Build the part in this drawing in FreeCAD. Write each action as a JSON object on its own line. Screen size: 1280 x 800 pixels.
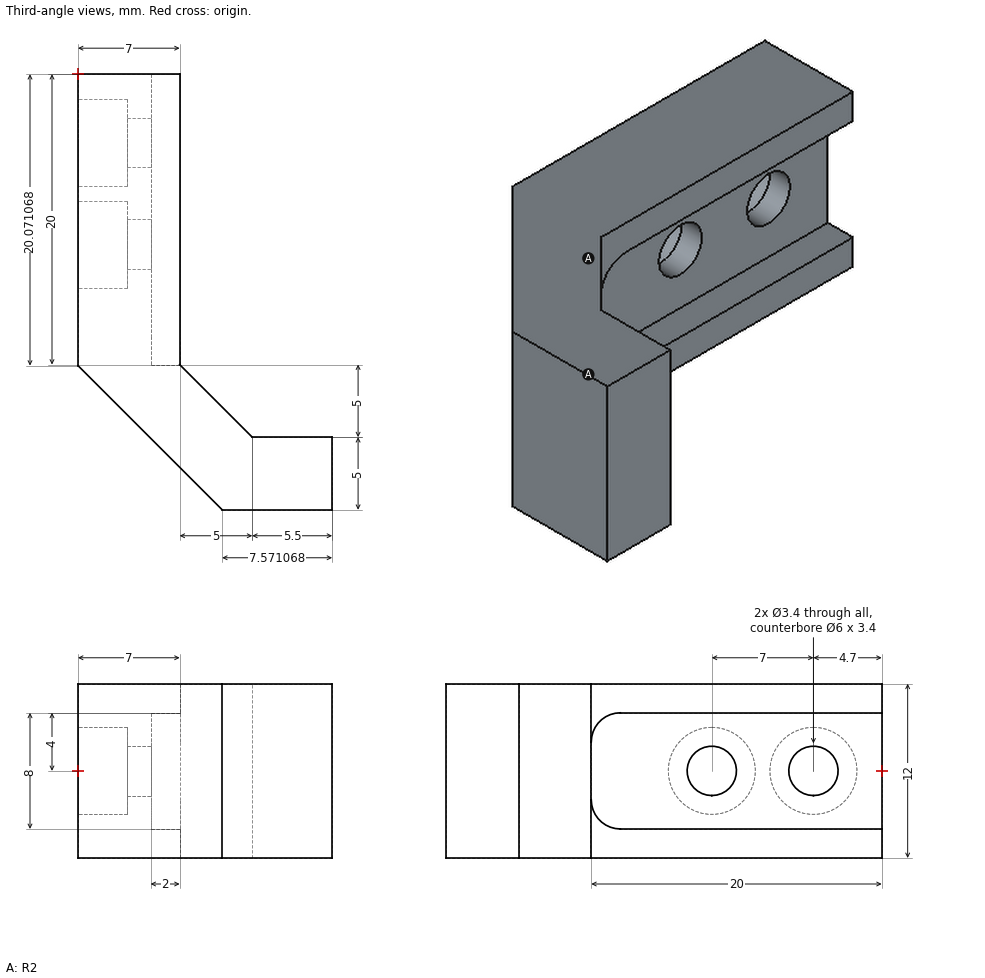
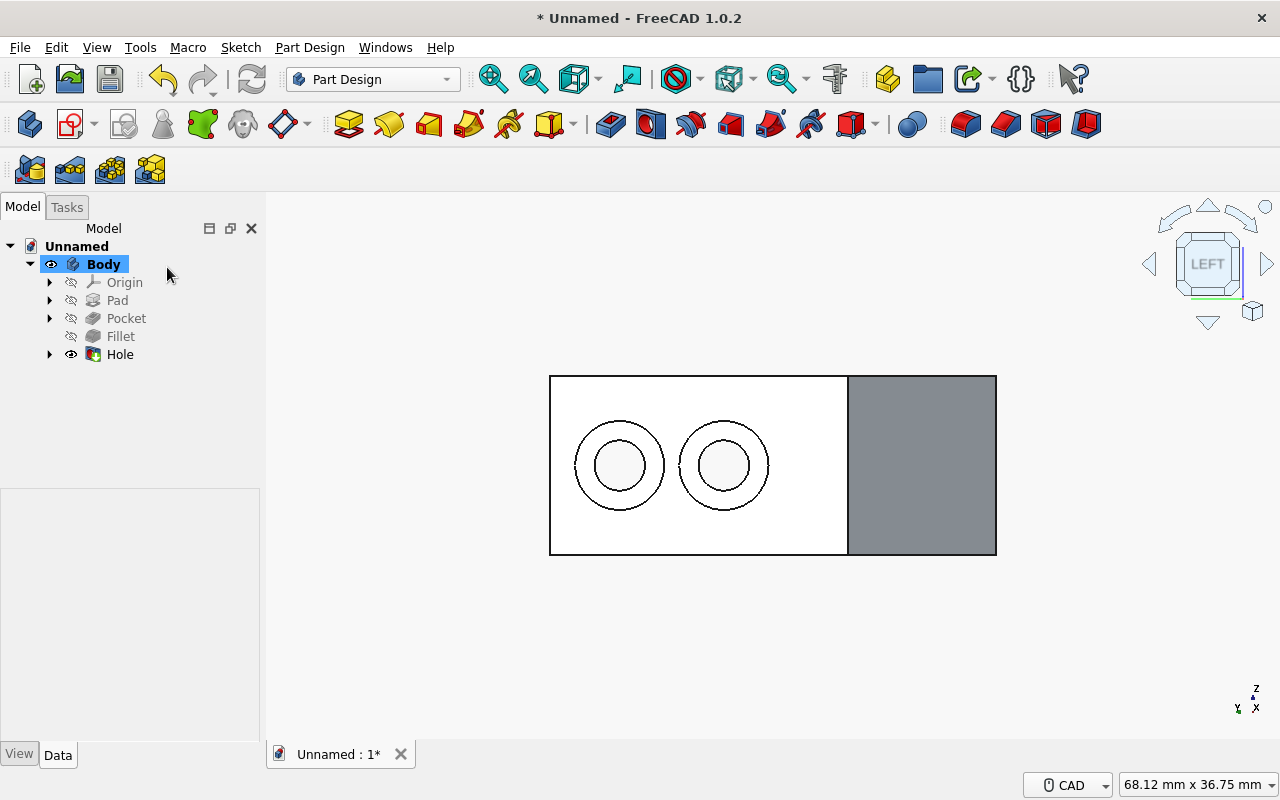
{"action": "key", "text": "0"}